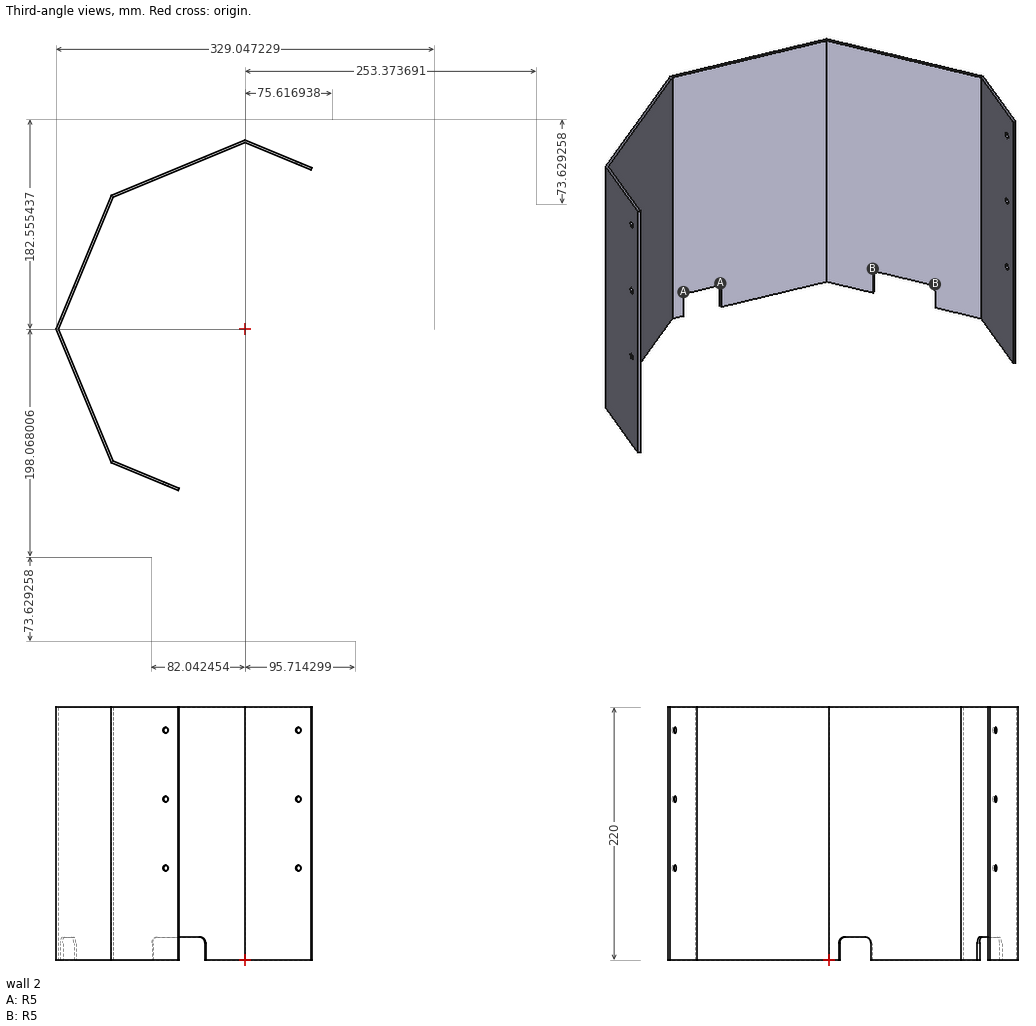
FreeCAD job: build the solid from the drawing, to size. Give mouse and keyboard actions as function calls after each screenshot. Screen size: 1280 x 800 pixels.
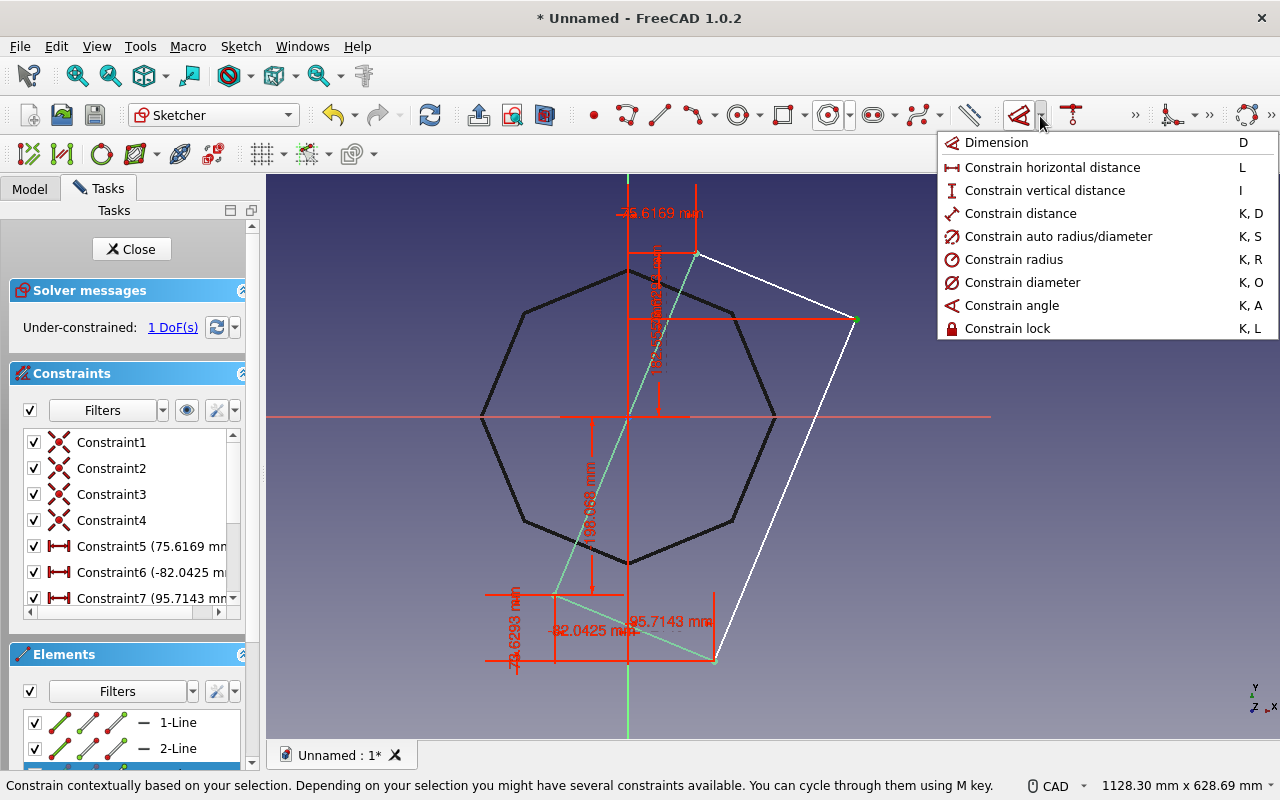
click(1108, 168)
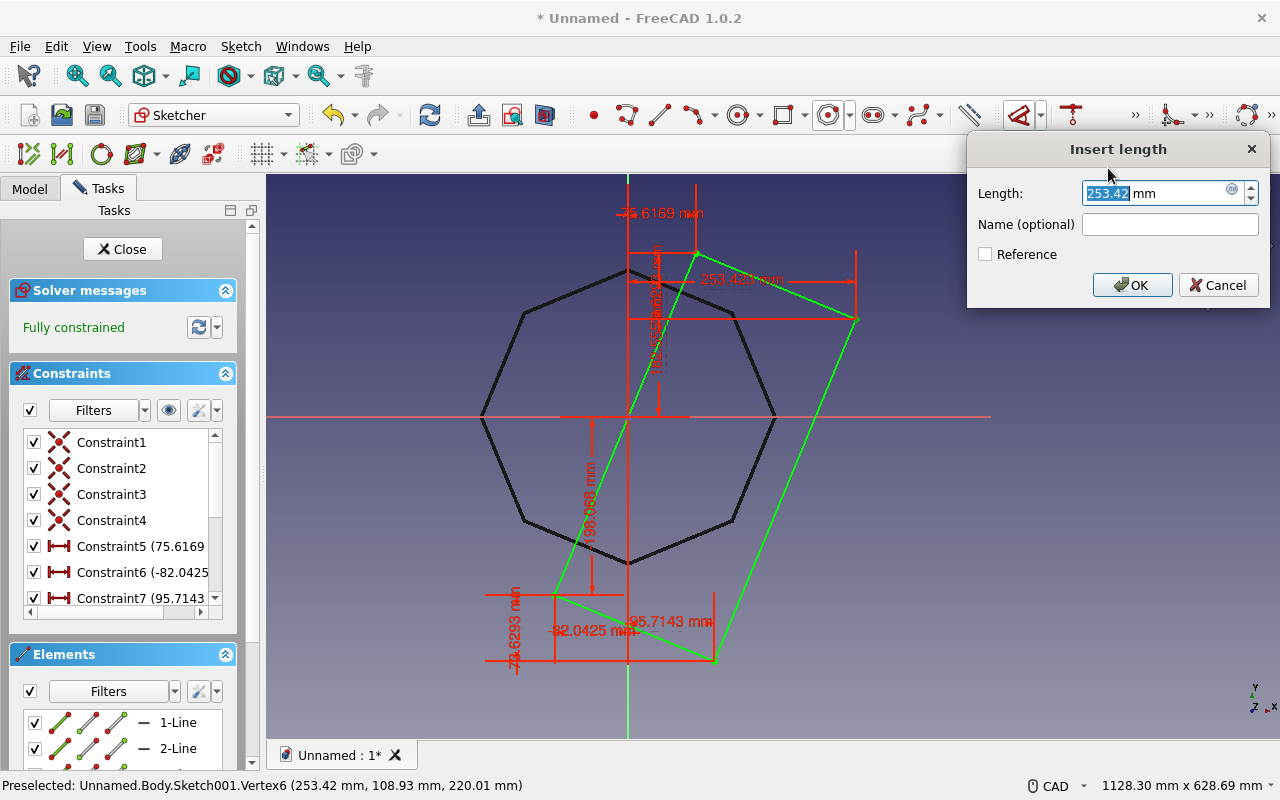
text(253.373691)
key(Return)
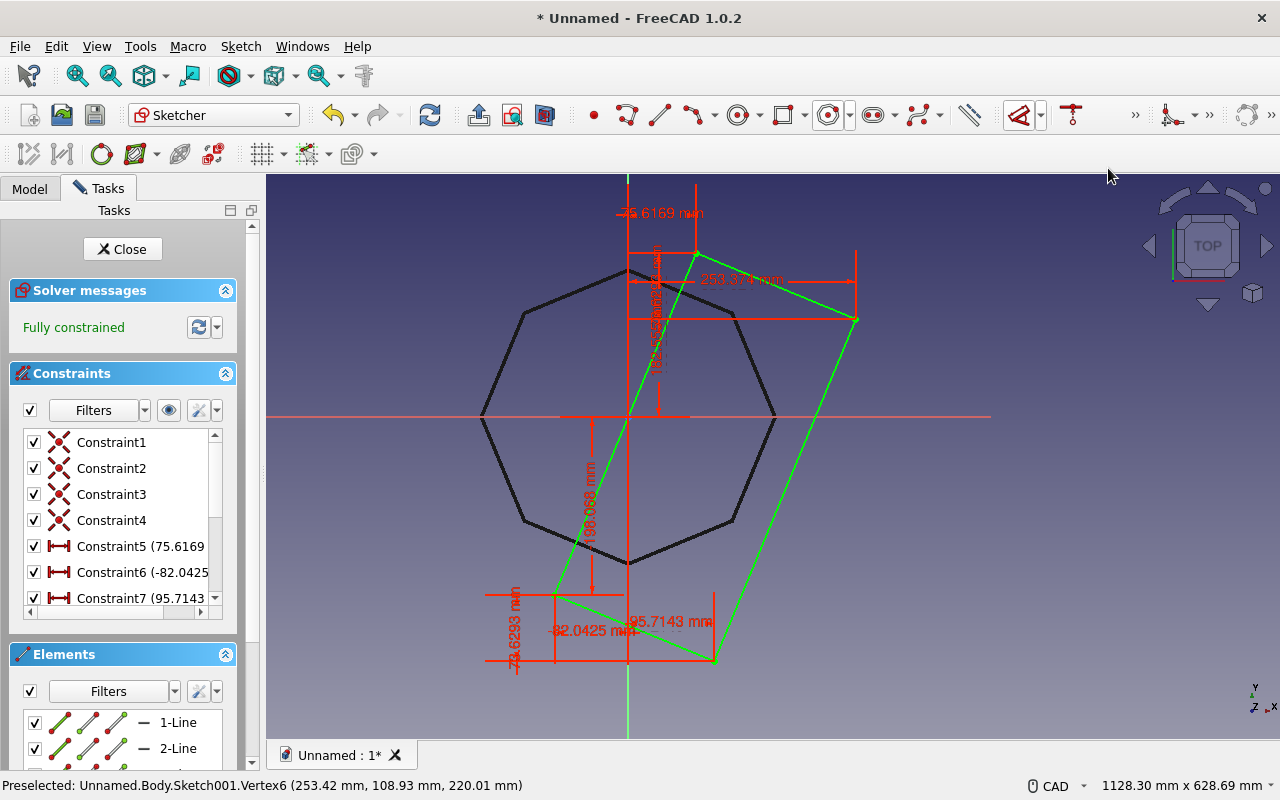
click(123, 249)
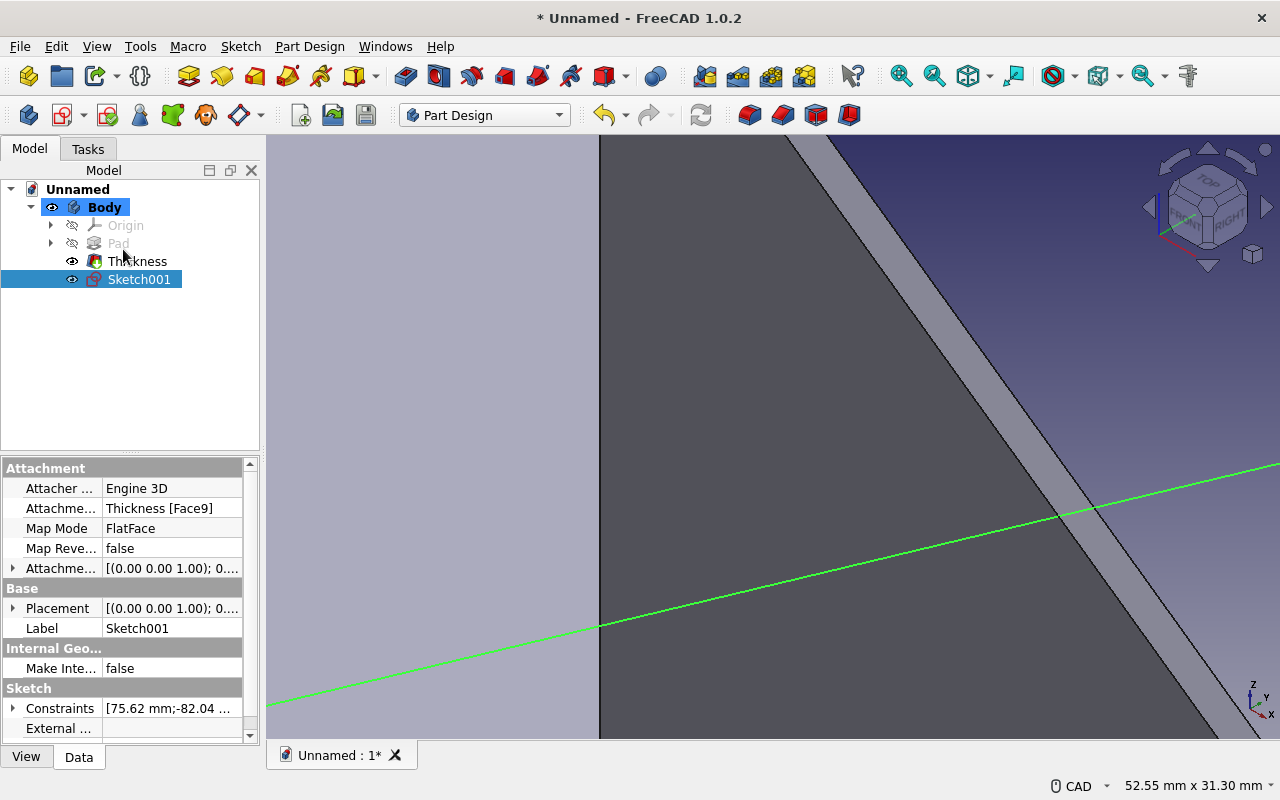
click(406, 76)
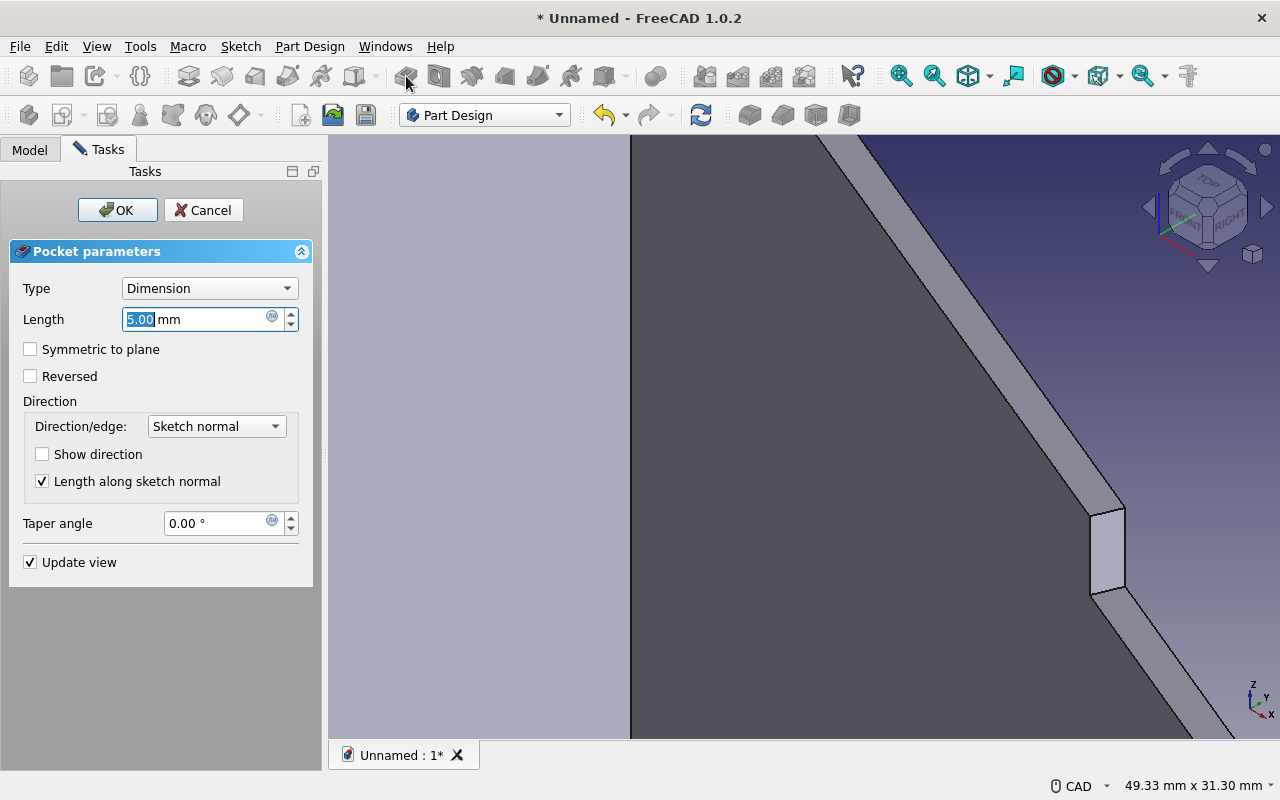
click(210, 288)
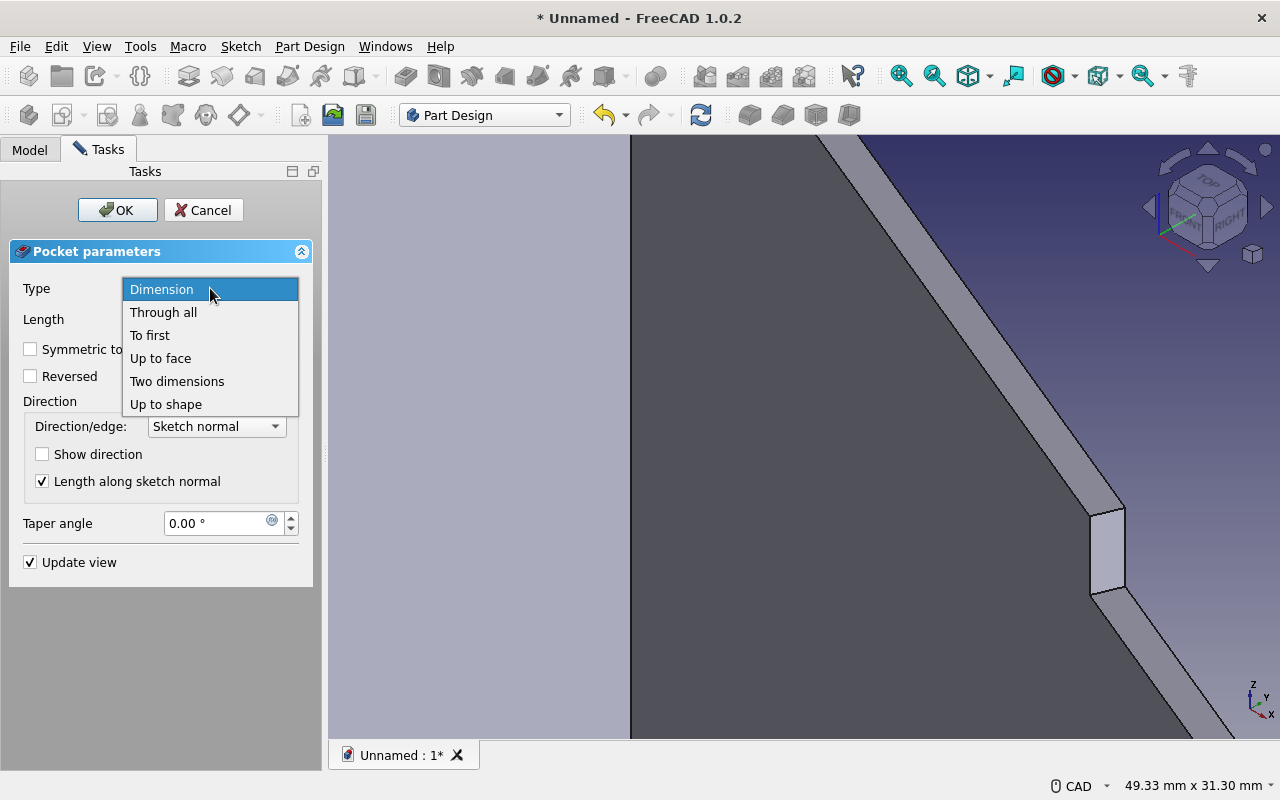
click(208, 312)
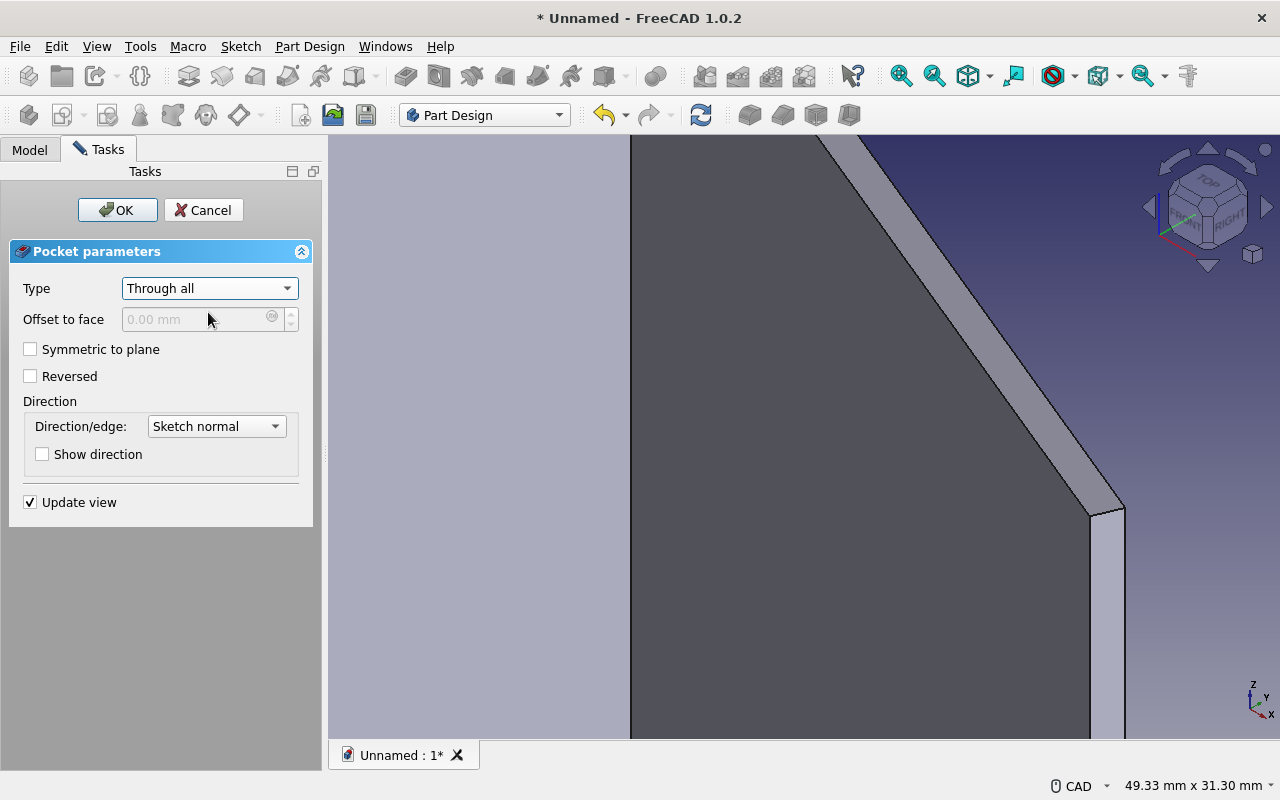
click(118, 210)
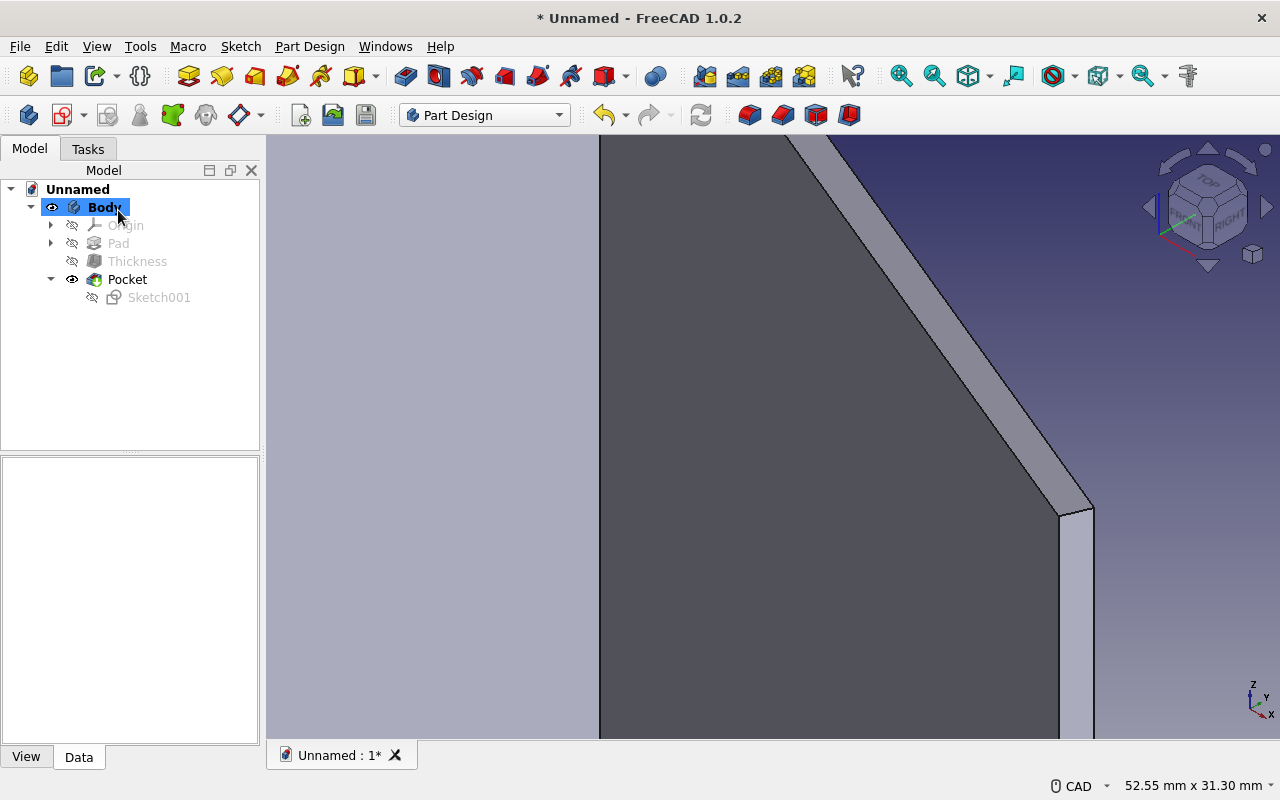
click(902, 76)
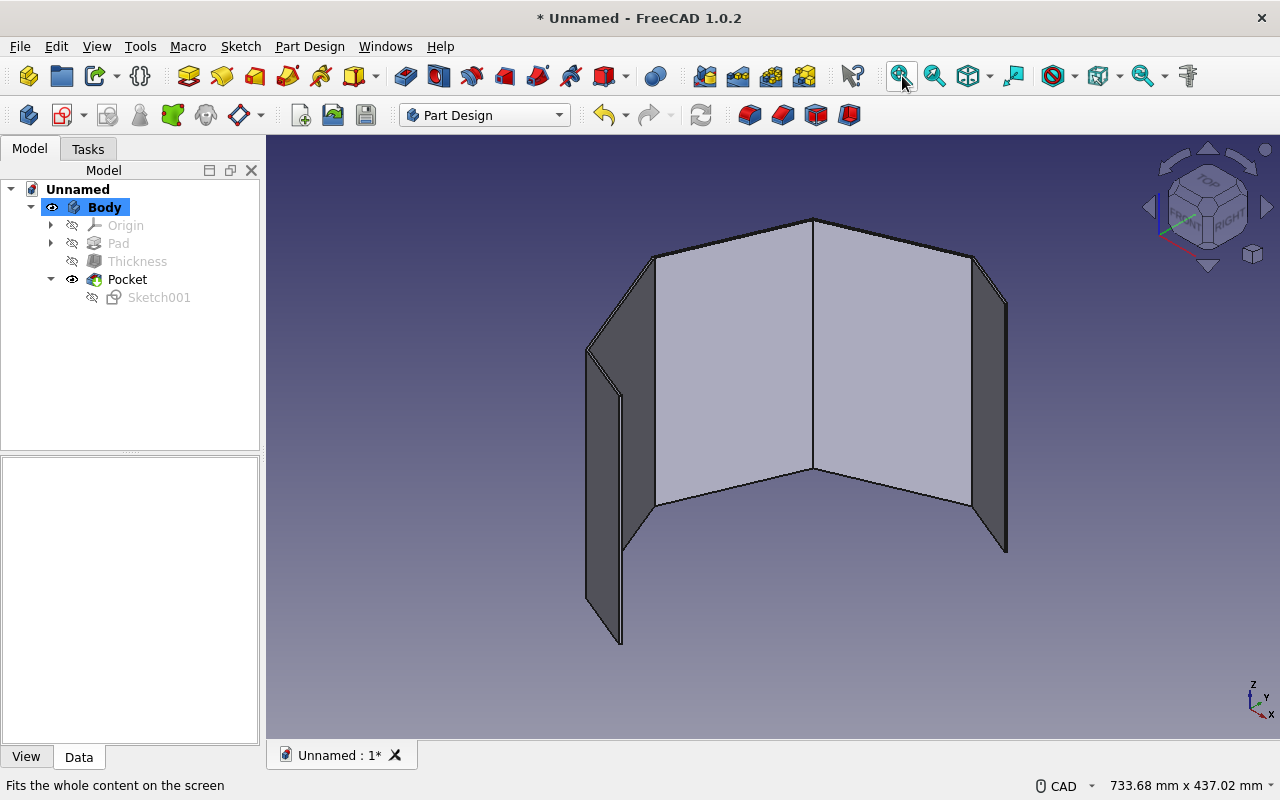
click(602, 425)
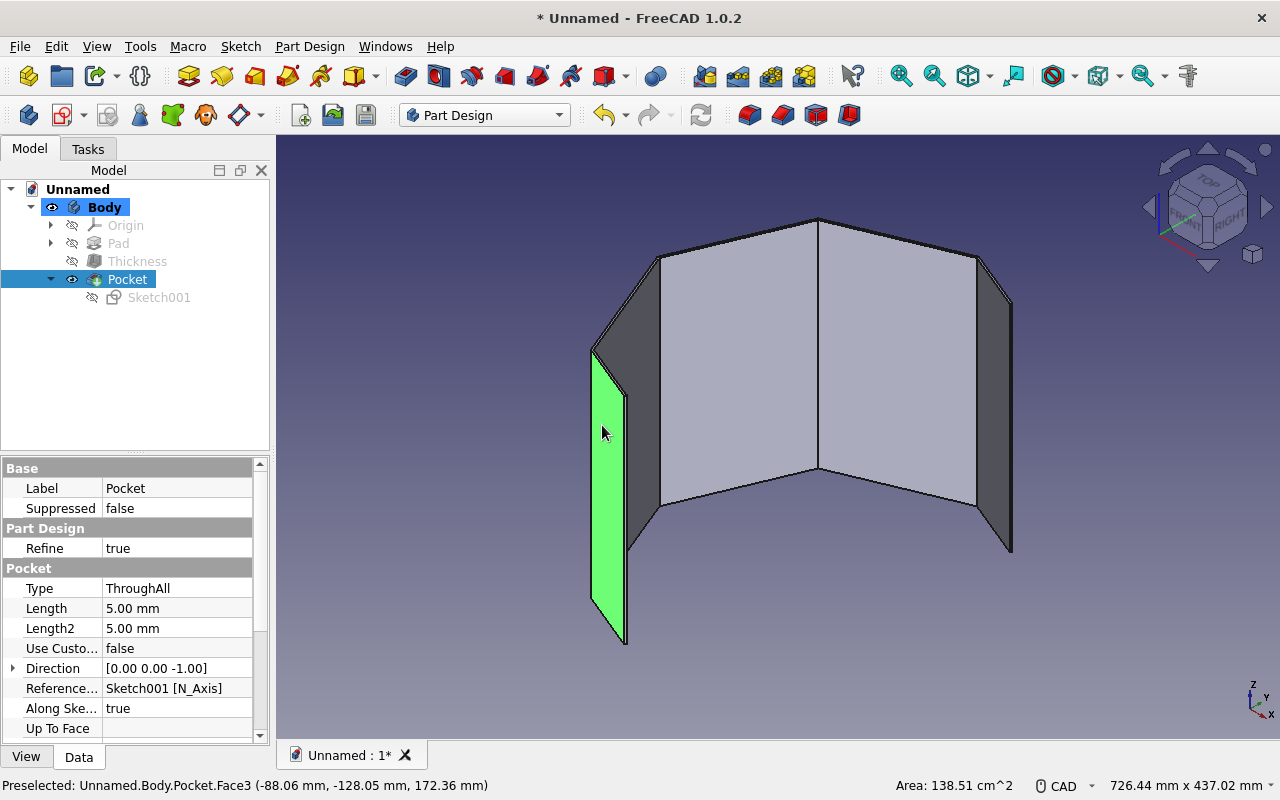
click(62, 116)